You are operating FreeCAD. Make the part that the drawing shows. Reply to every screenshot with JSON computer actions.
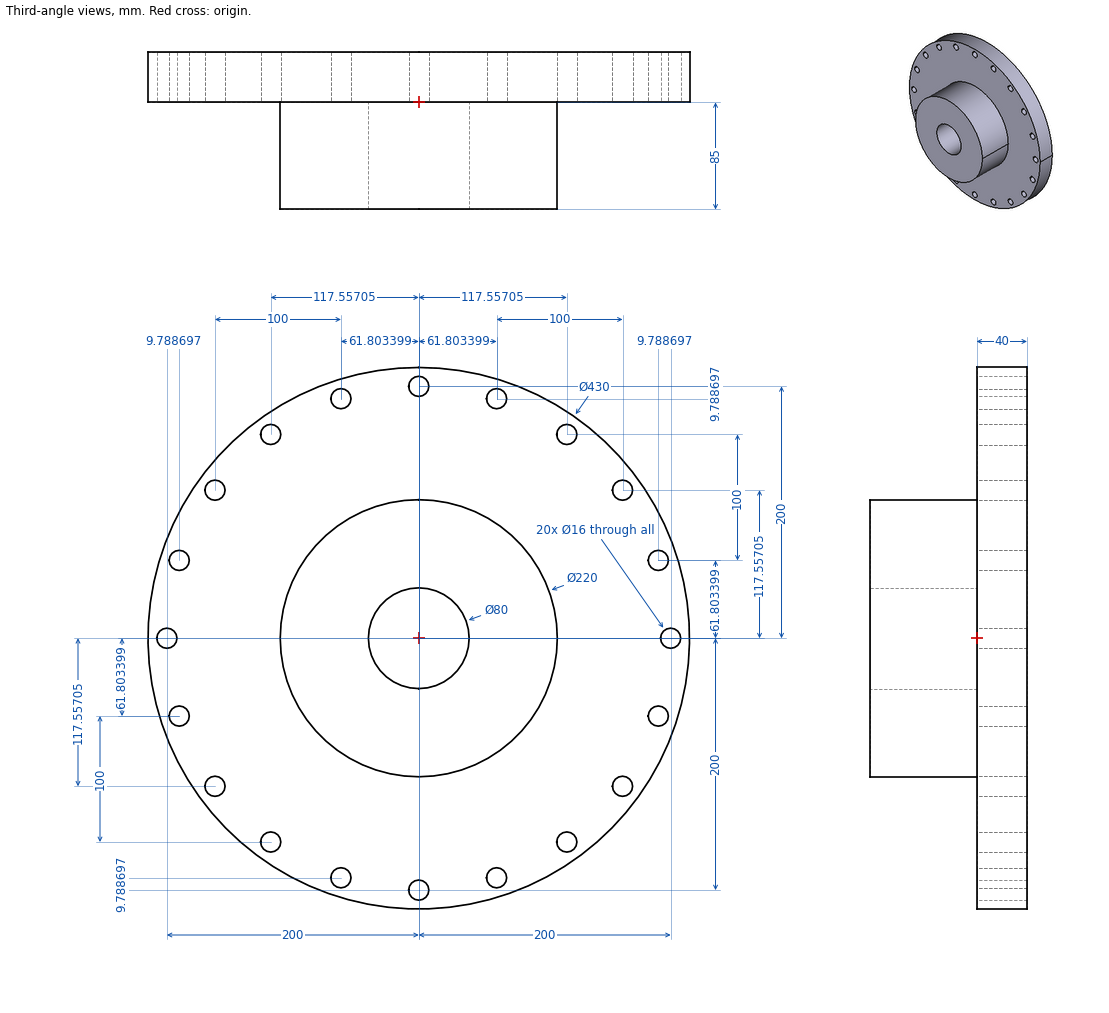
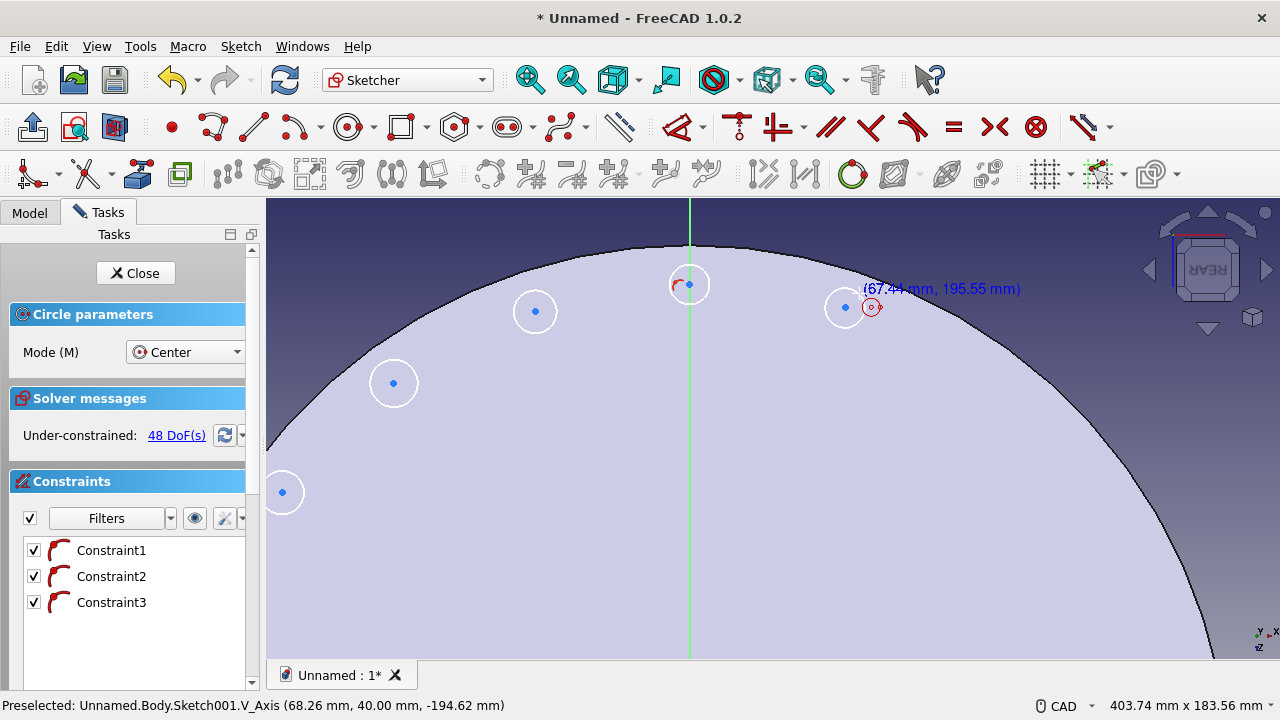
{"action": "left_click", "coordinate": [985, 379]}
{"action": "left_click", "coordinate": [999, 365]}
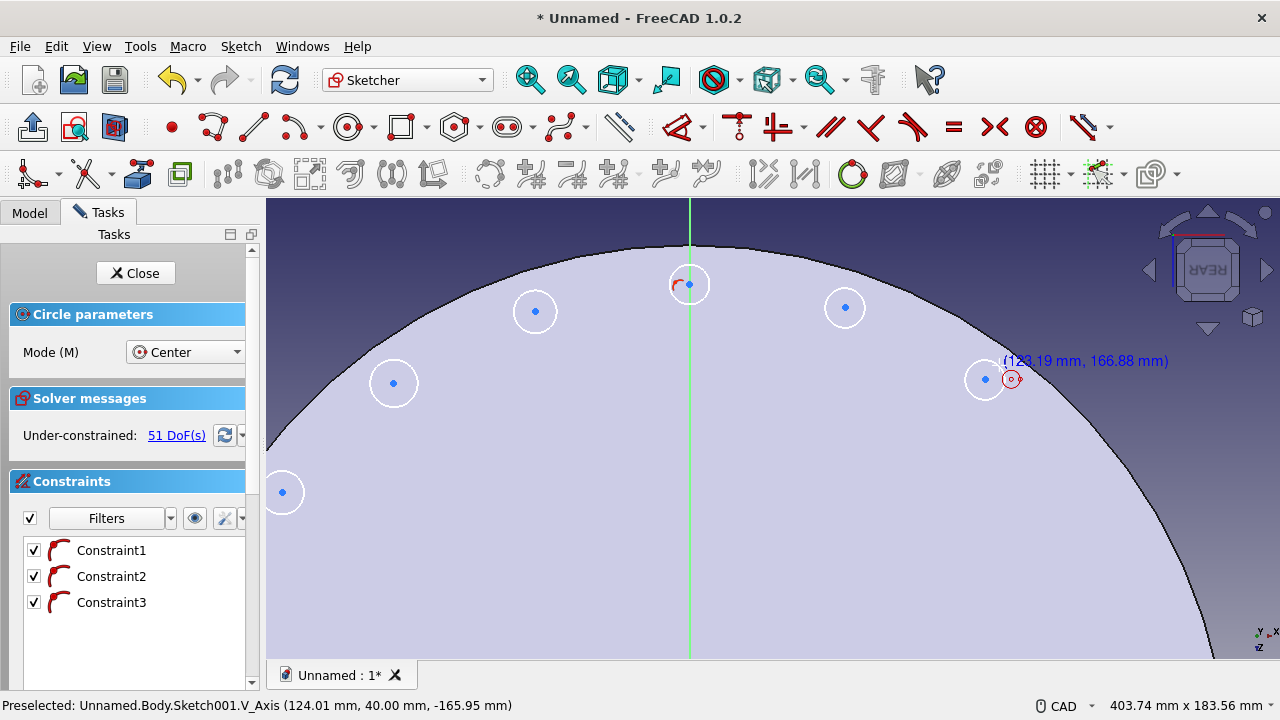
{"action": "left_click", "coordinate": [1096, 490]}
{"action": "left_click", "coordinate": [1110, 476]}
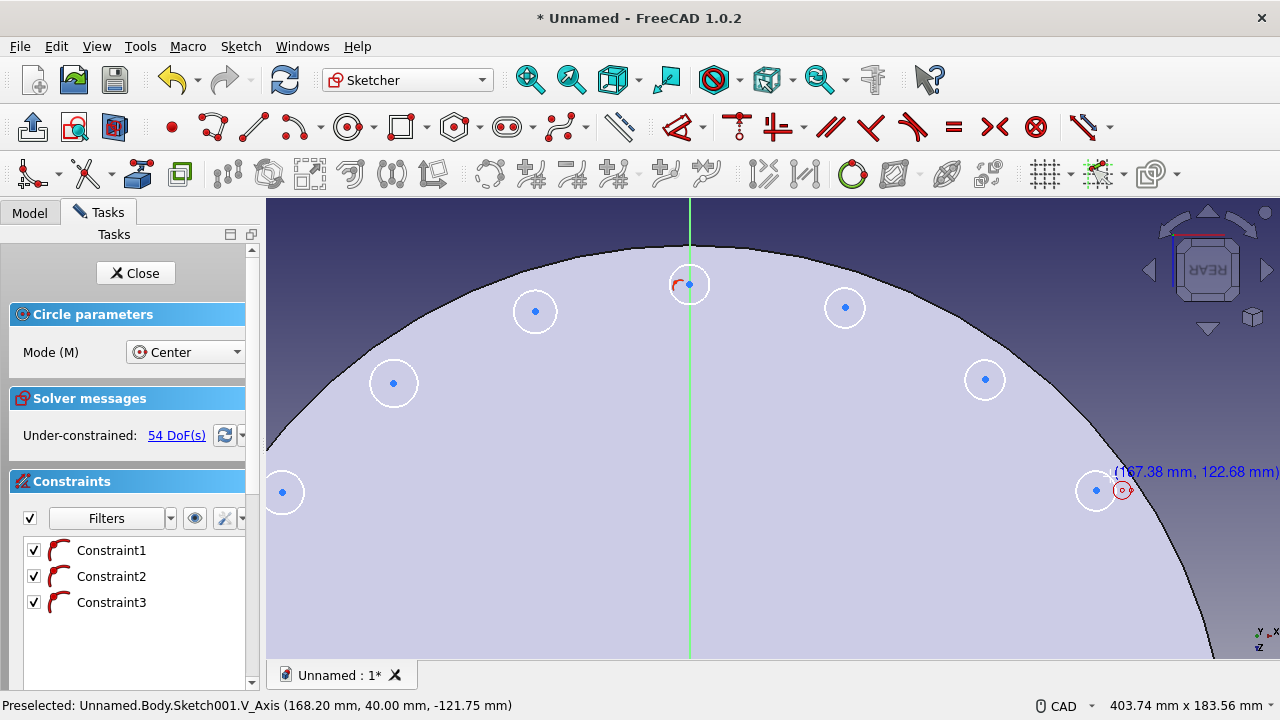
{"action": "scroll", "coordinate": [711, 275], "scroll_direction": "down", "scroll_amount": 6}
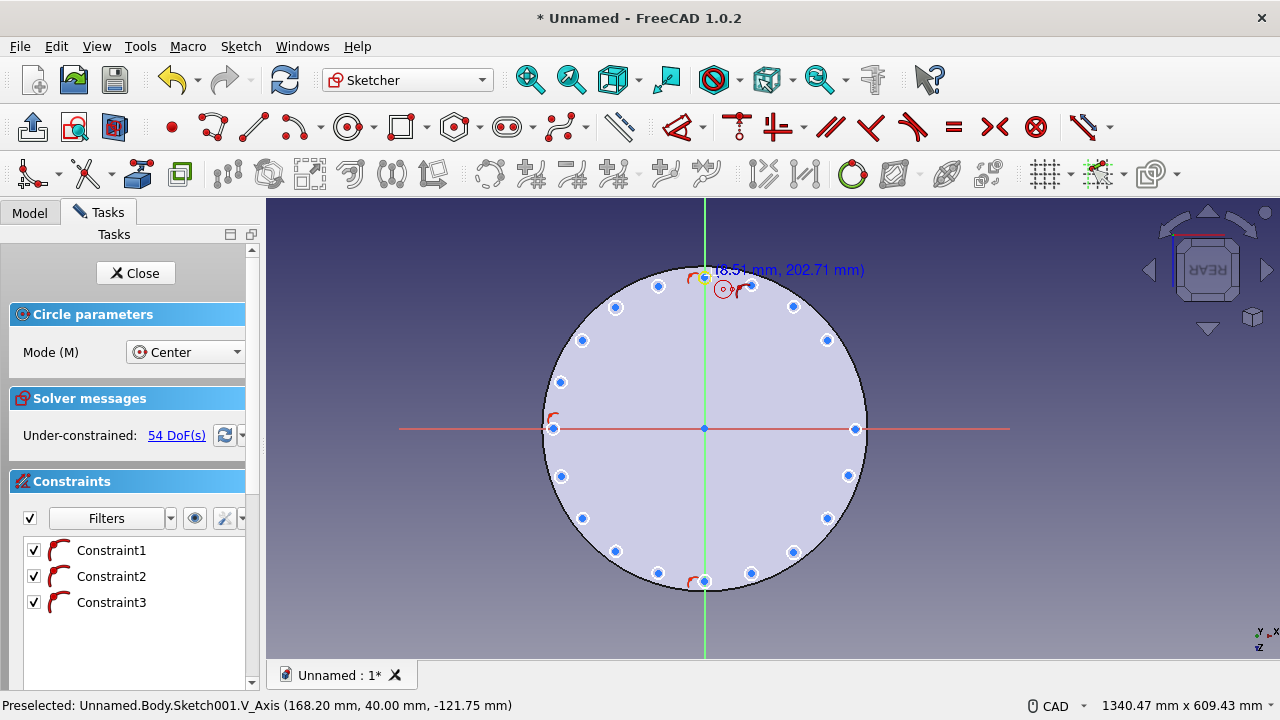
{"action": "scroll", "coordinate": [849, 382], "scroll_direction": "up", "scroll_amount": 7}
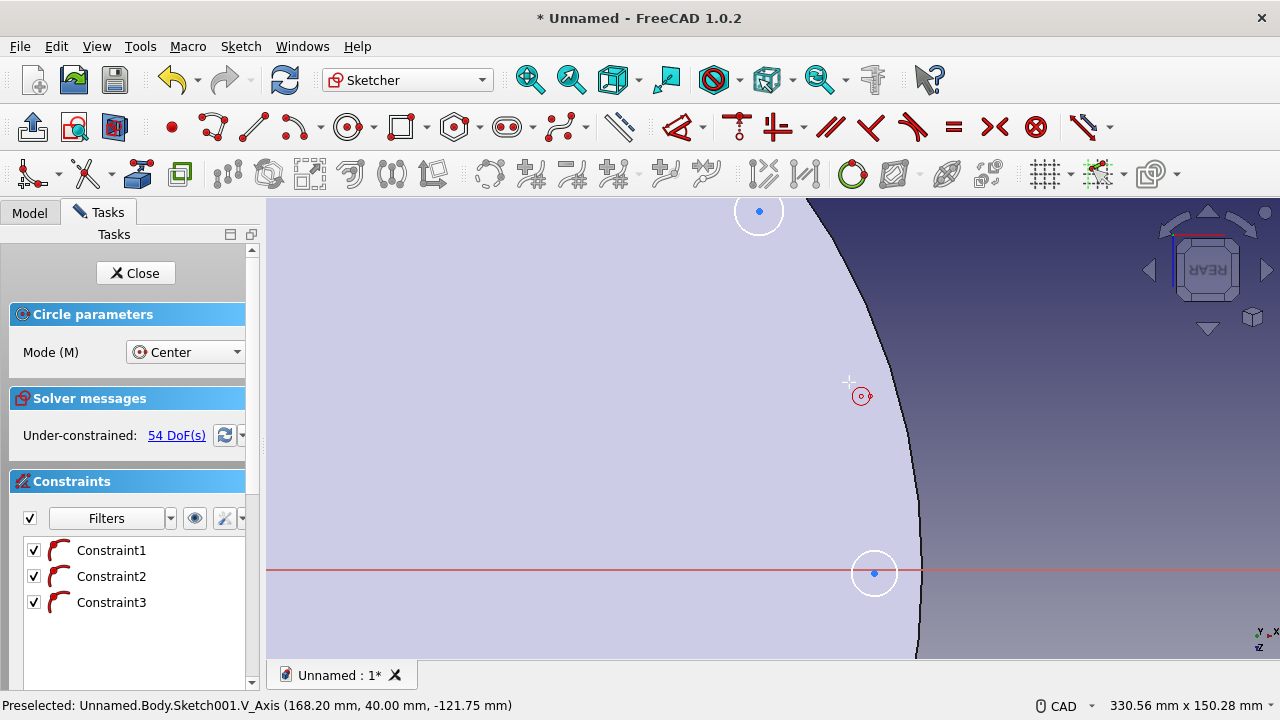
{"action": "scroll", "coordinate": [849, 382], "scroll_direction": "down", "scroll_amount": 7}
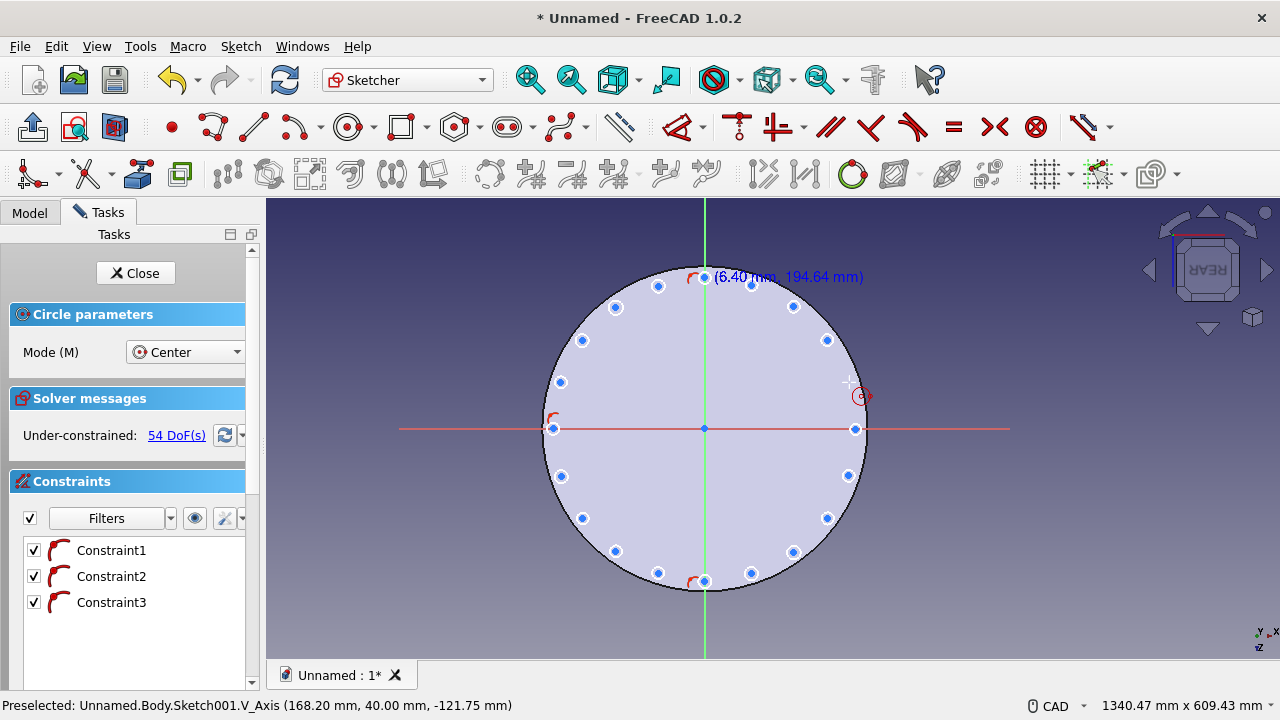
{"action": "left_click", "coordinate": [849, 382]}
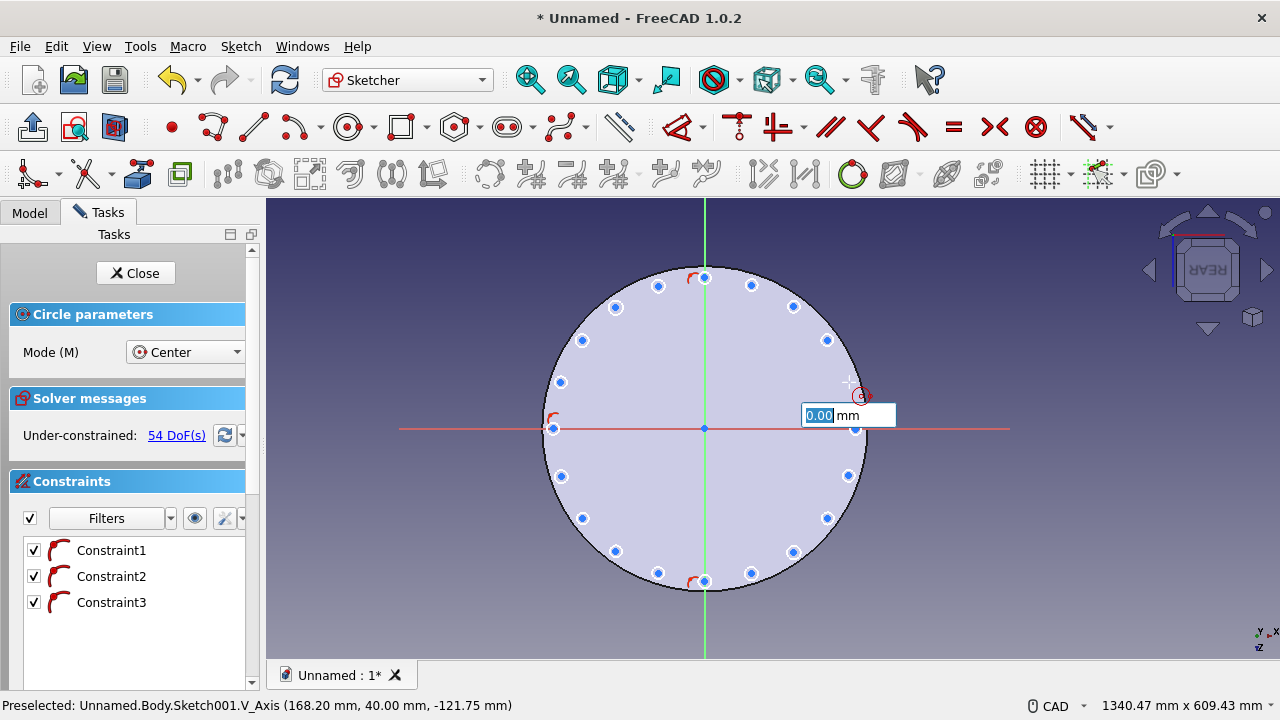
{"action": "scroll", "coordinate": [853, 378], "scroll_direction": "up", "scroll_amount": 5}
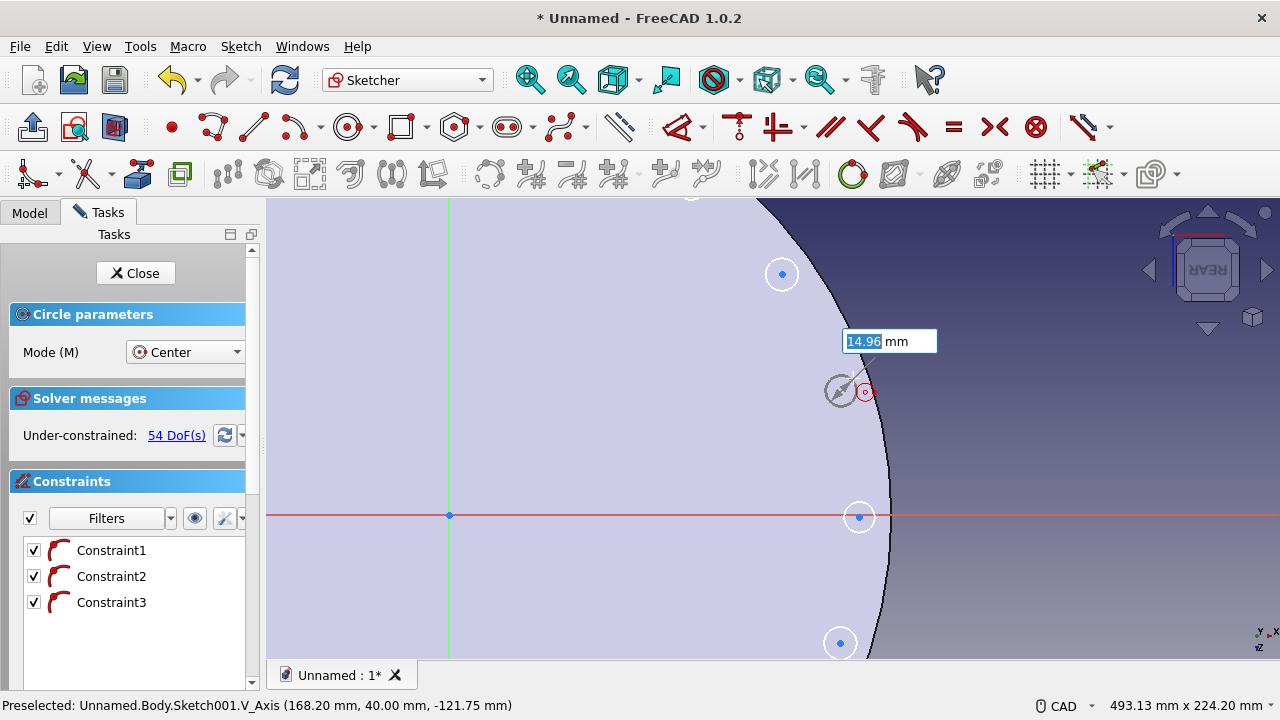
{"action": "left_click", "coordinate": [852, 377]}
{"action": "key", "text": "Escape"}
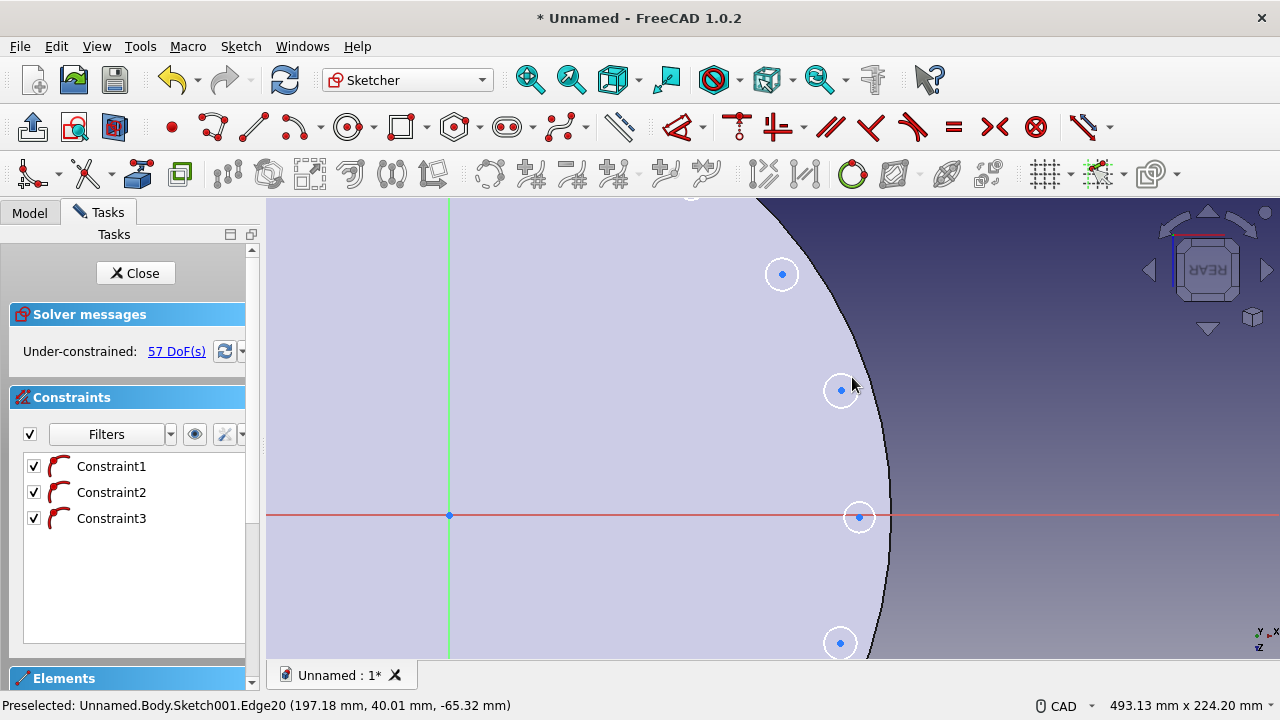
{"action": "left_click", "coordinate": [849, 528]}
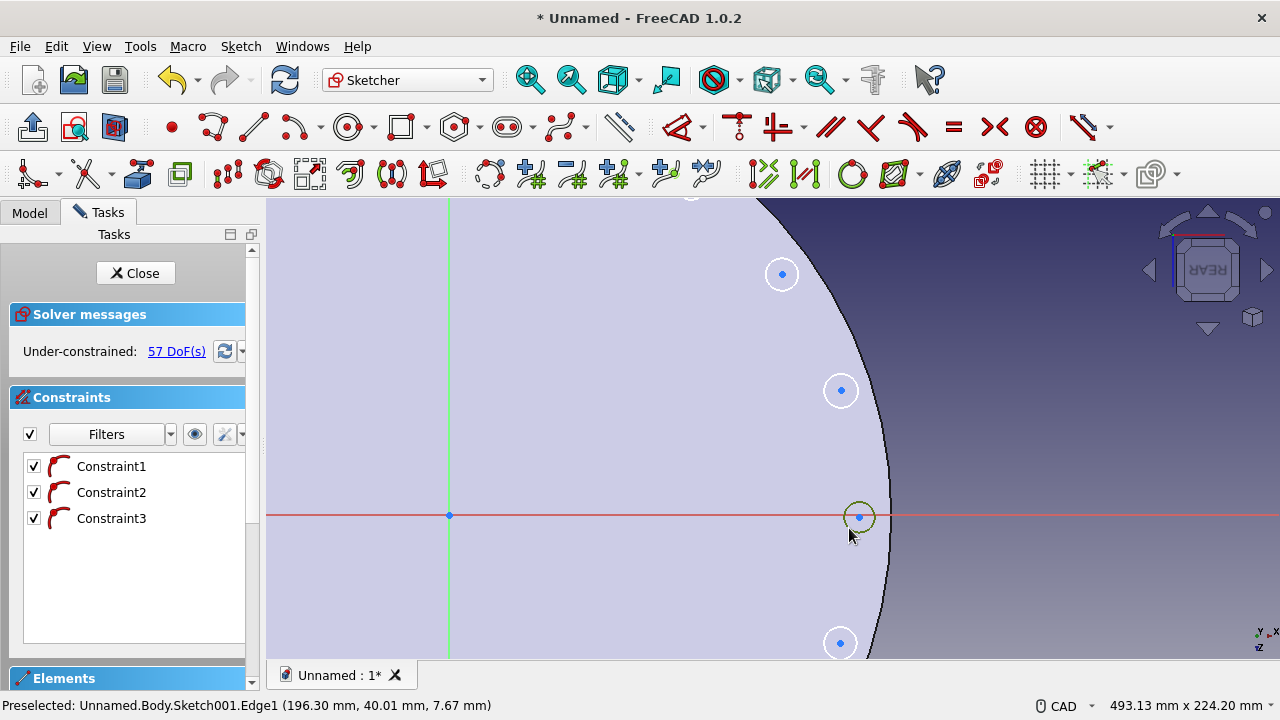
{"action": "left_click", "coordinate": [841, 627]}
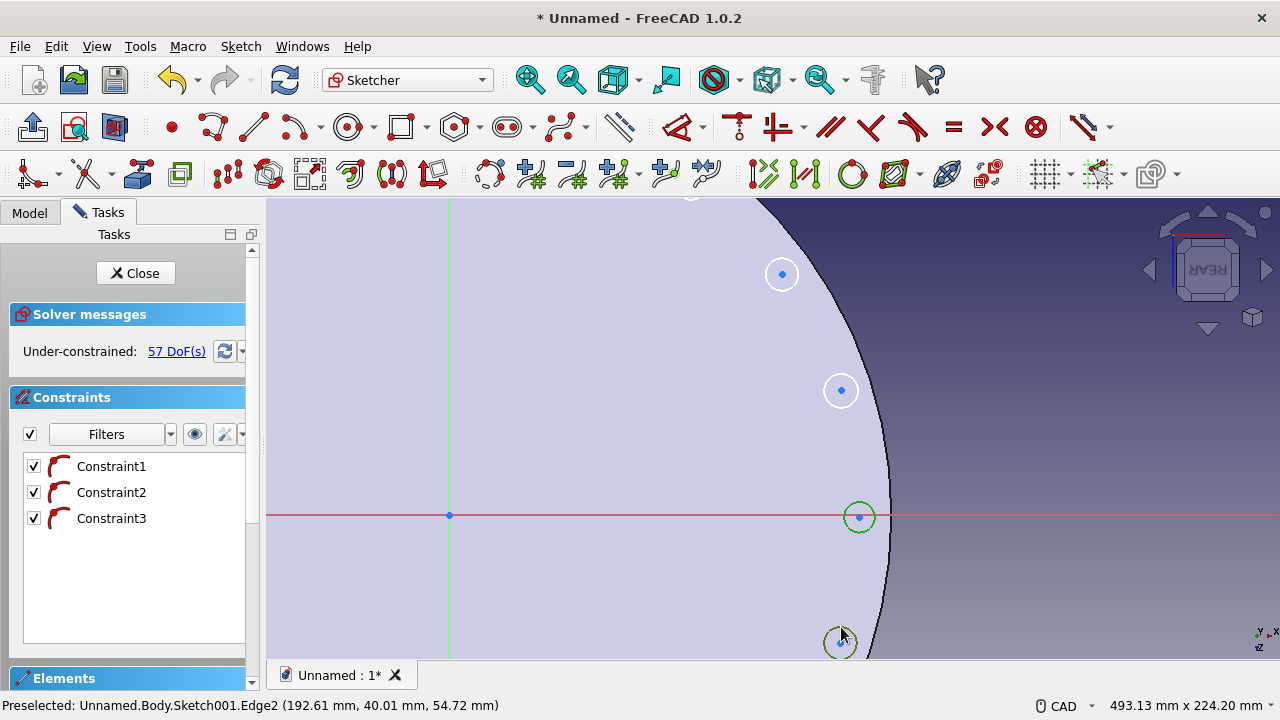
{"action": "scroll", "coordinate": [853, 378], "scroll_direction": "down", "scroll_amount": 5}